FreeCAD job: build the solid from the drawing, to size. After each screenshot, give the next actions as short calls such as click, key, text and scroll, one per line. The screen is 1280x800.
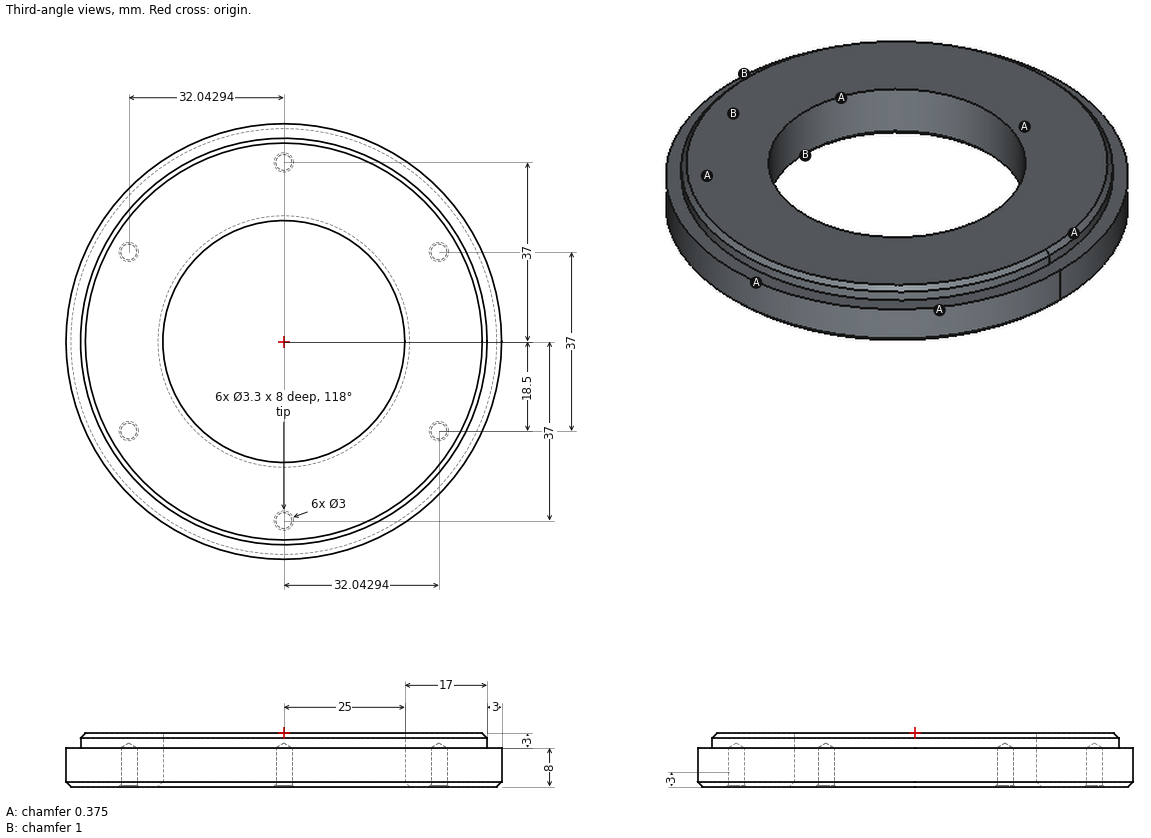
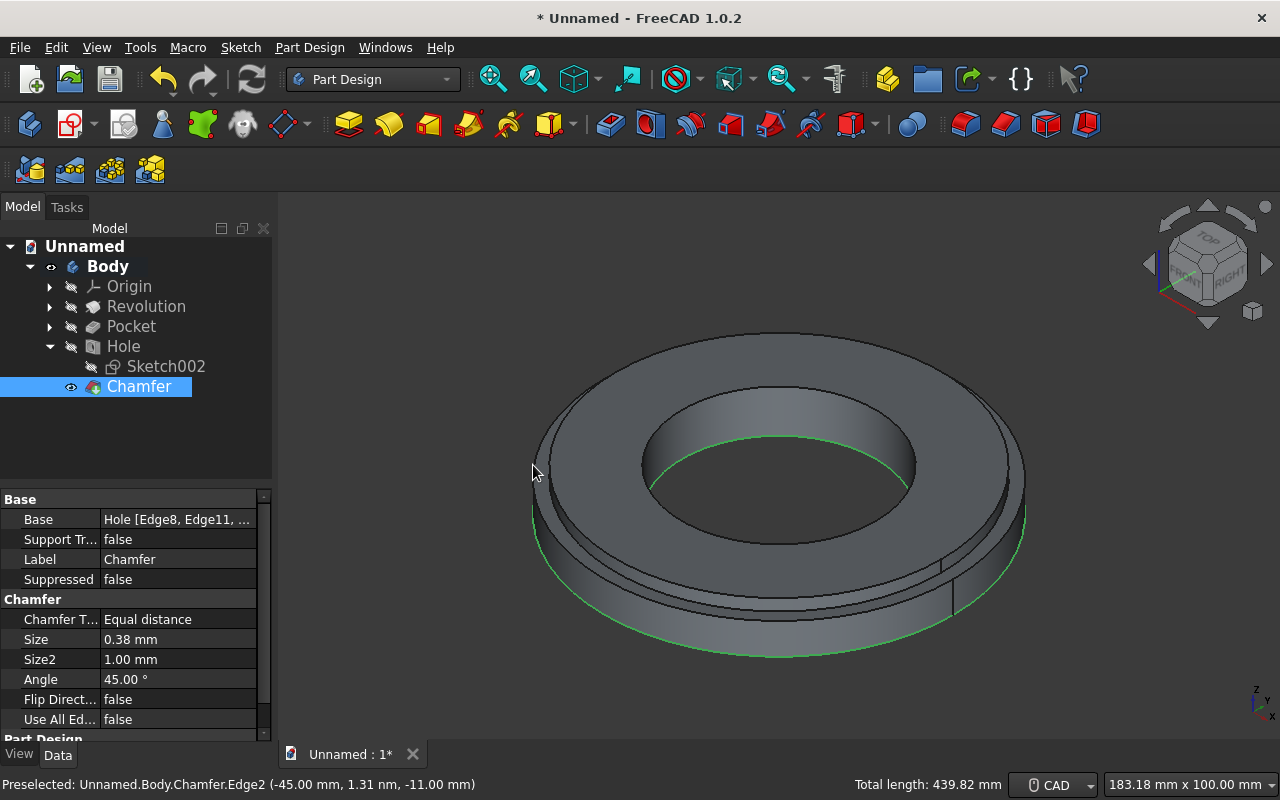
click(574, 525, ctrl)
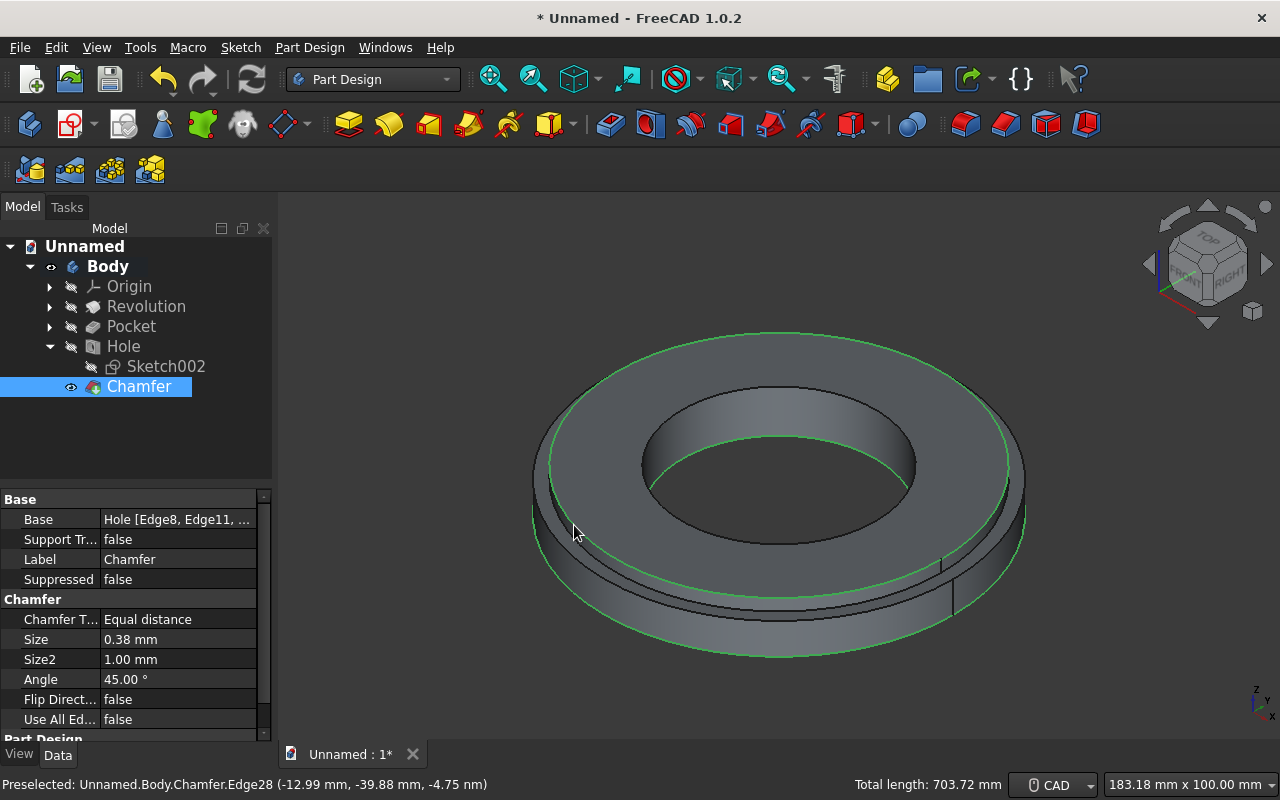
click(1006, 124)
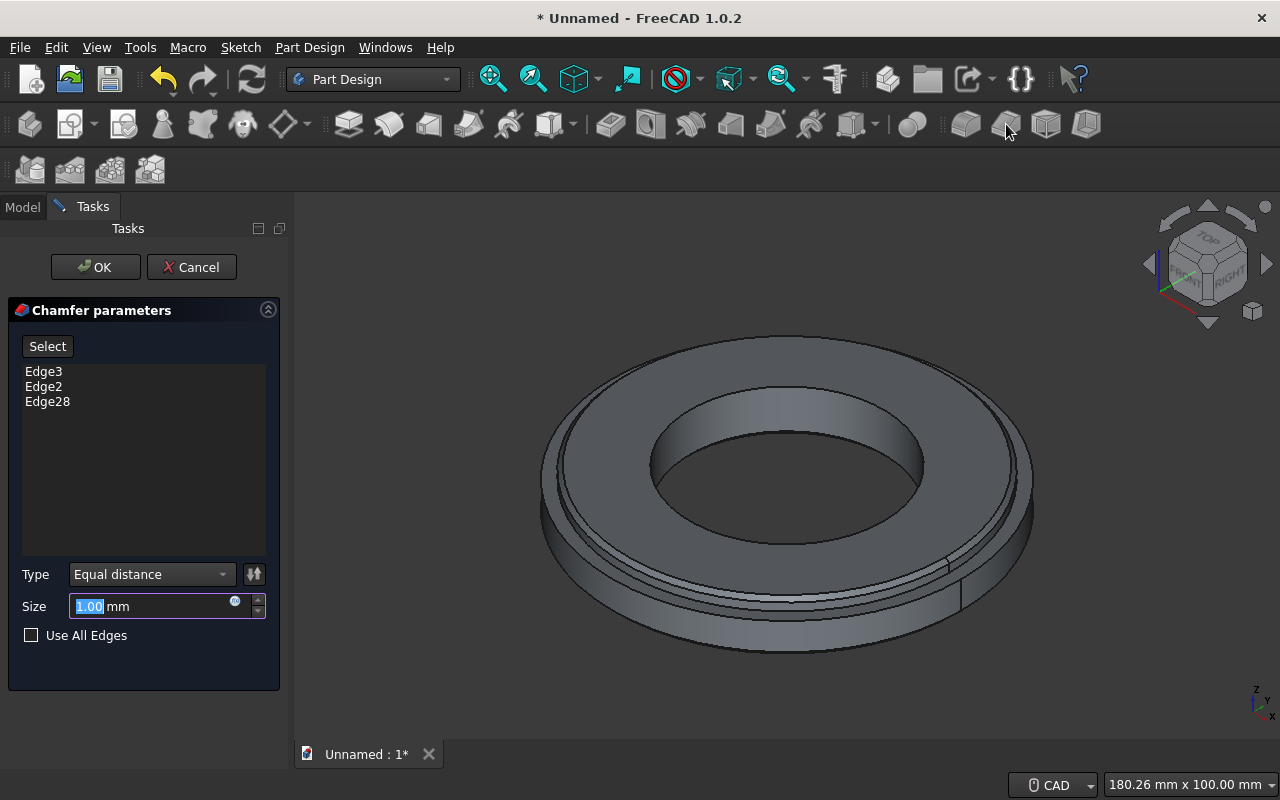
text(1)
key(Tab)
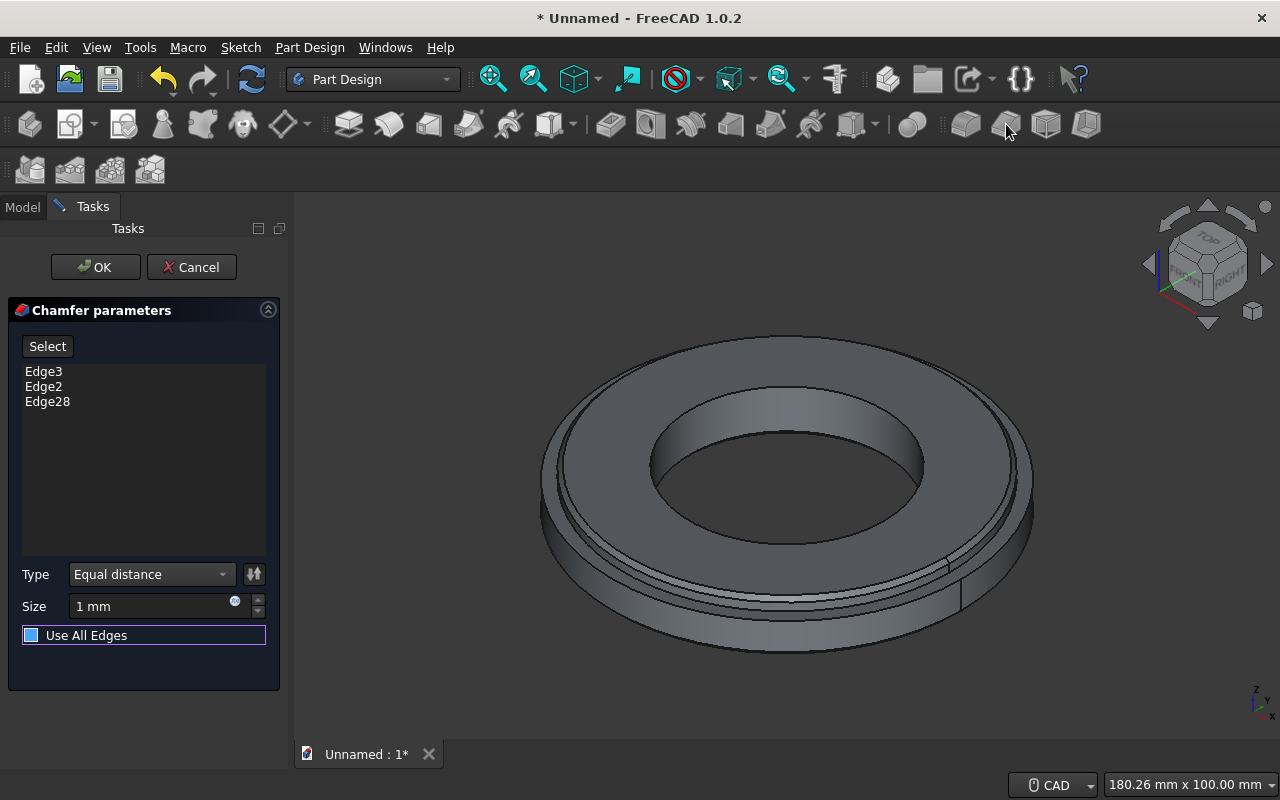
click(96, 267)